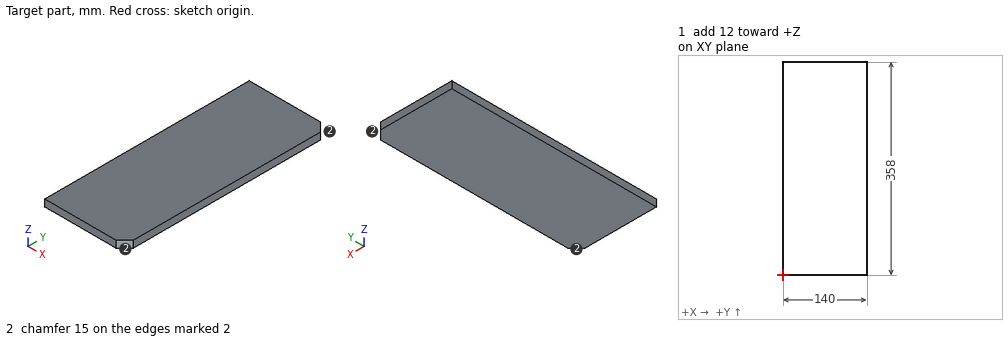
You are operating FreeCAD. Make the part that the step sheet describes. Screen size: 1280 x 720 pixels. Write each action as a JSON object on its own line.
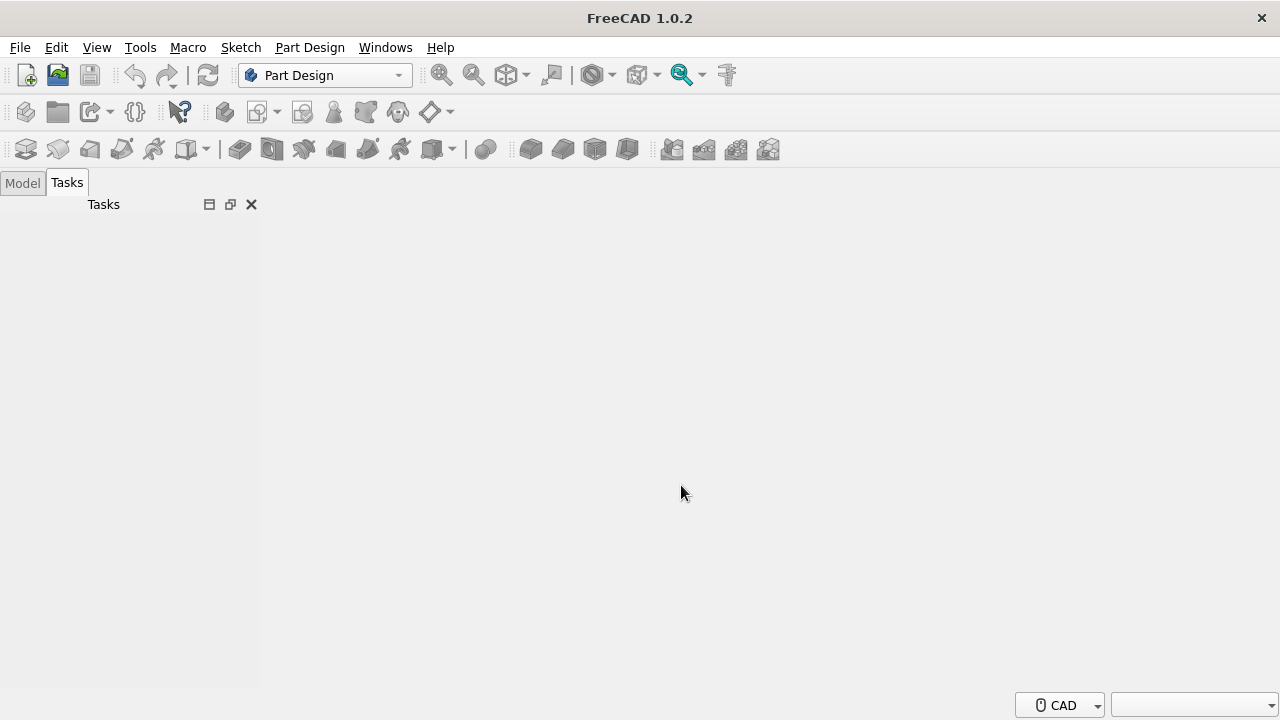
{"action": "left_click", "coordinate": [26, 76]}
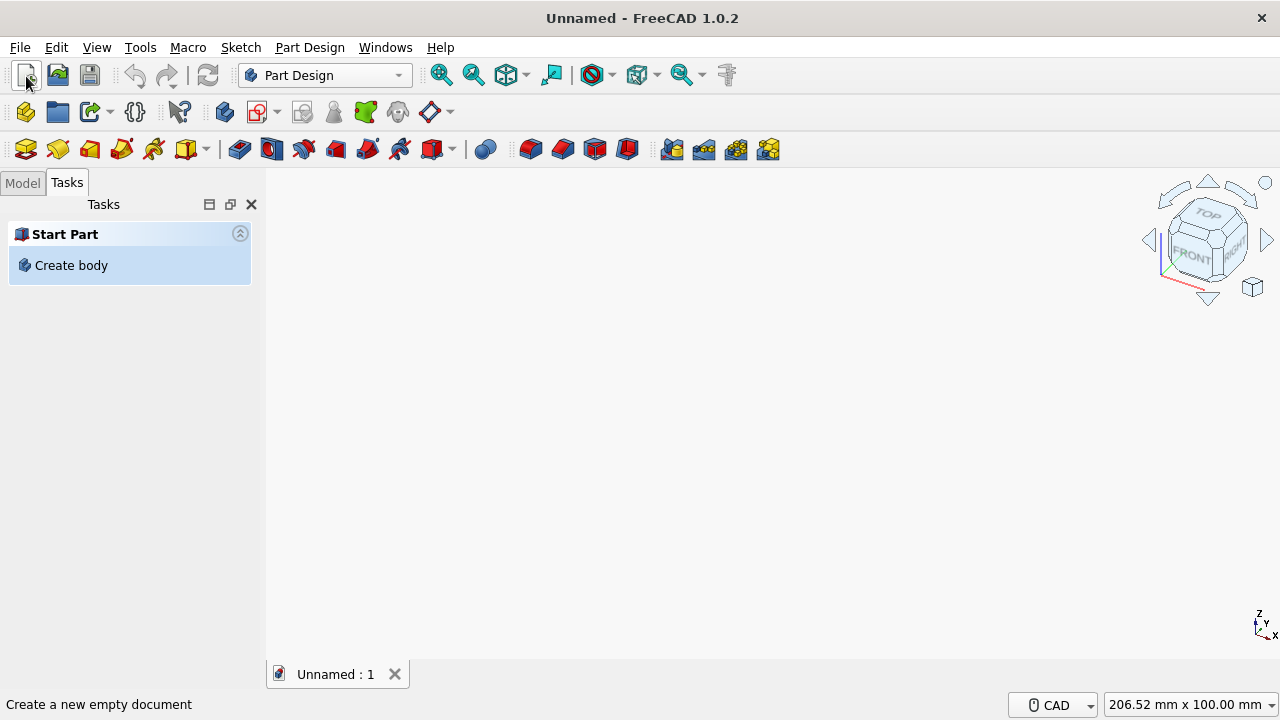
{"action": "left_click", "coordinate": [258, 112]}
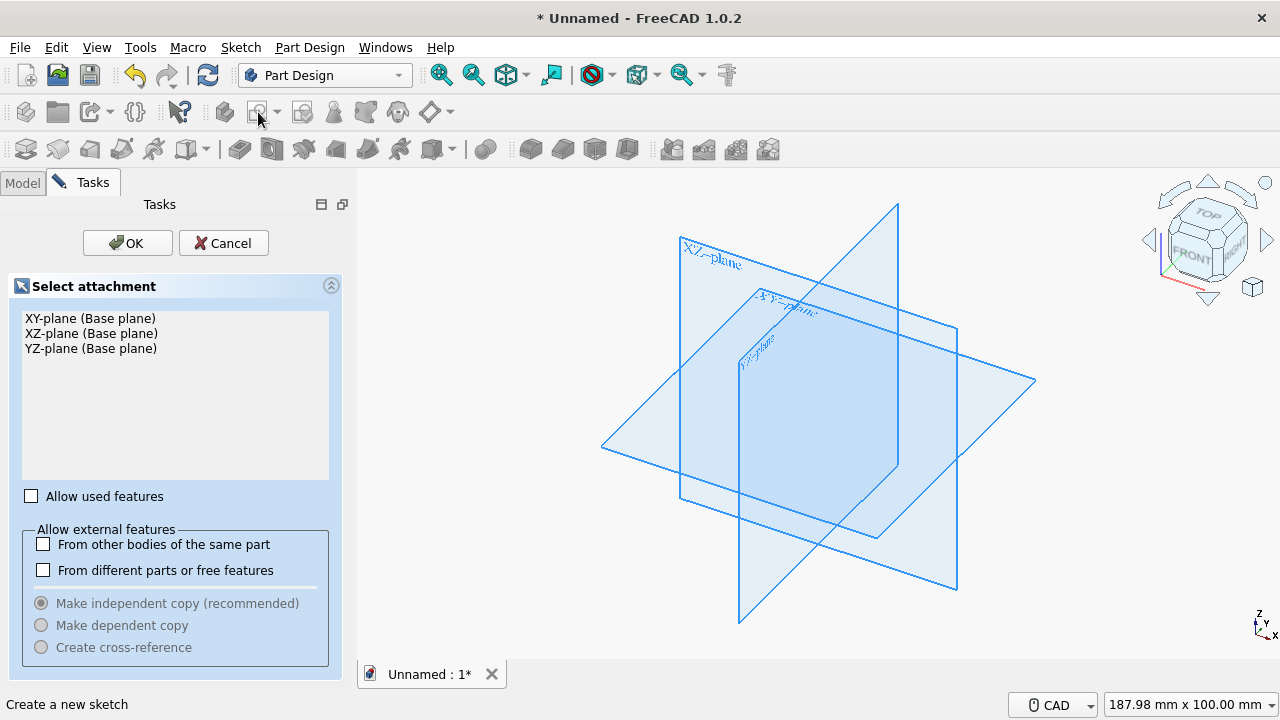
{"action": "left_click", "coordinate": [82, 318]}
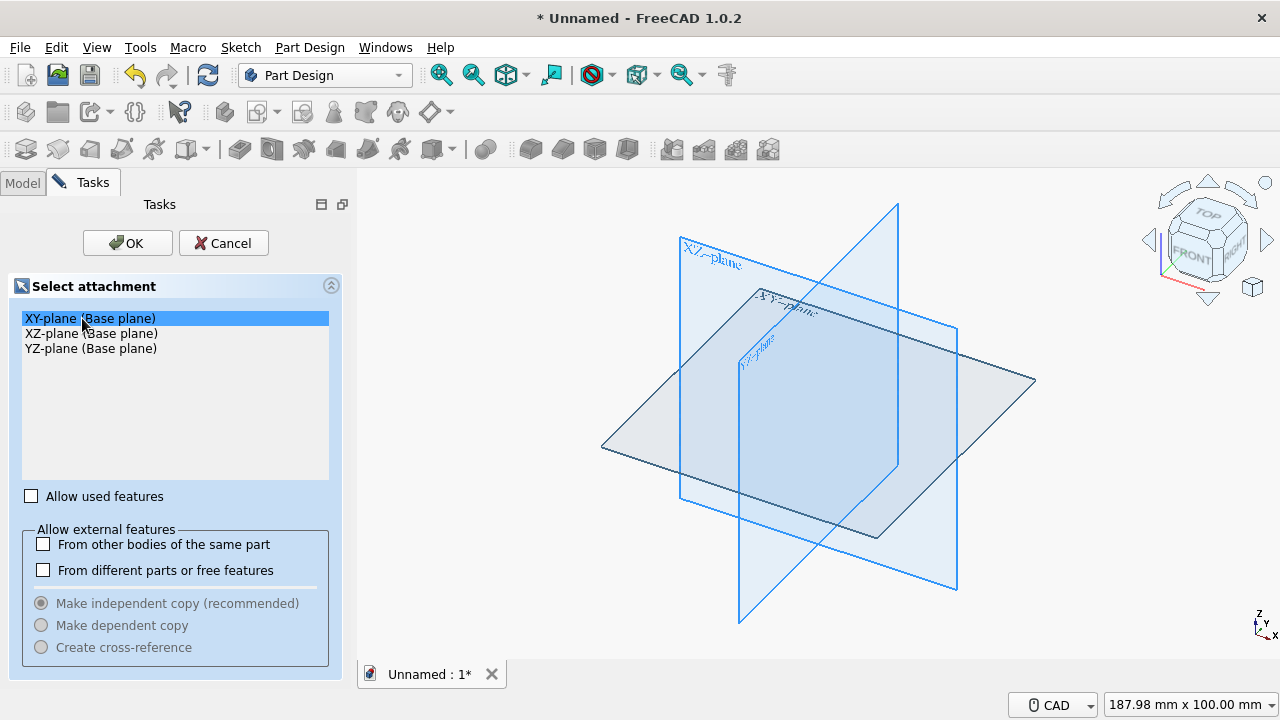
{"action": "left_click", "coordinate": [128, 243]}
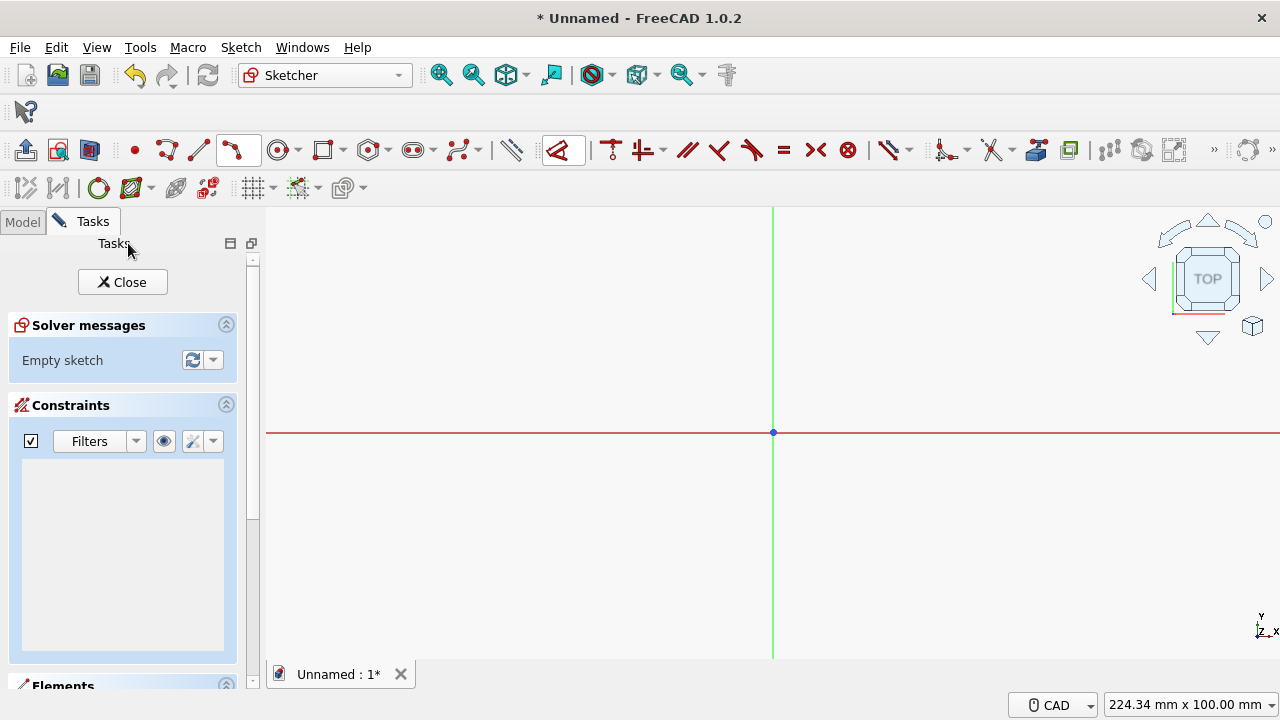
{"action": "scroll", "coordinate": [628, 593], "scroll_direction": "down", "scroll_amount": 9}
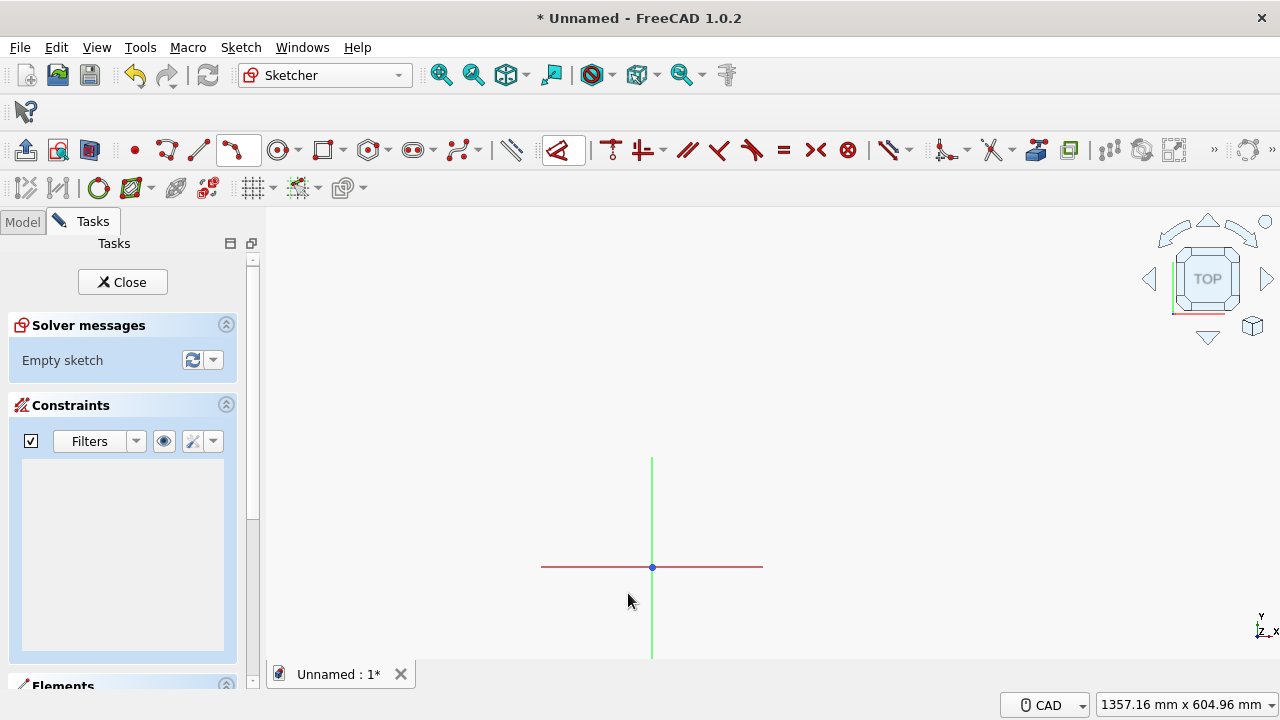
{"action": "left_click", "coordinate": [324, 150]}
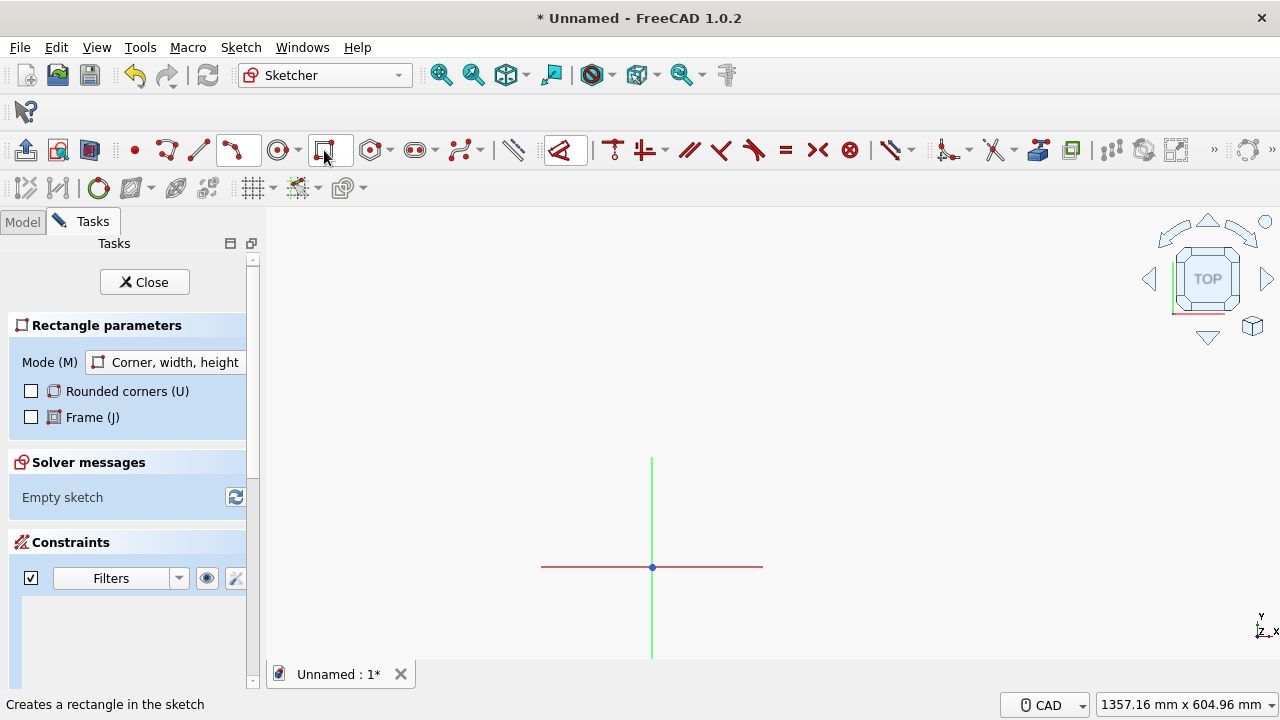
{"action": "left_click", "coordinate": [652, 567]}
{"action": "mouse_move", "coordinate": [757, 300]}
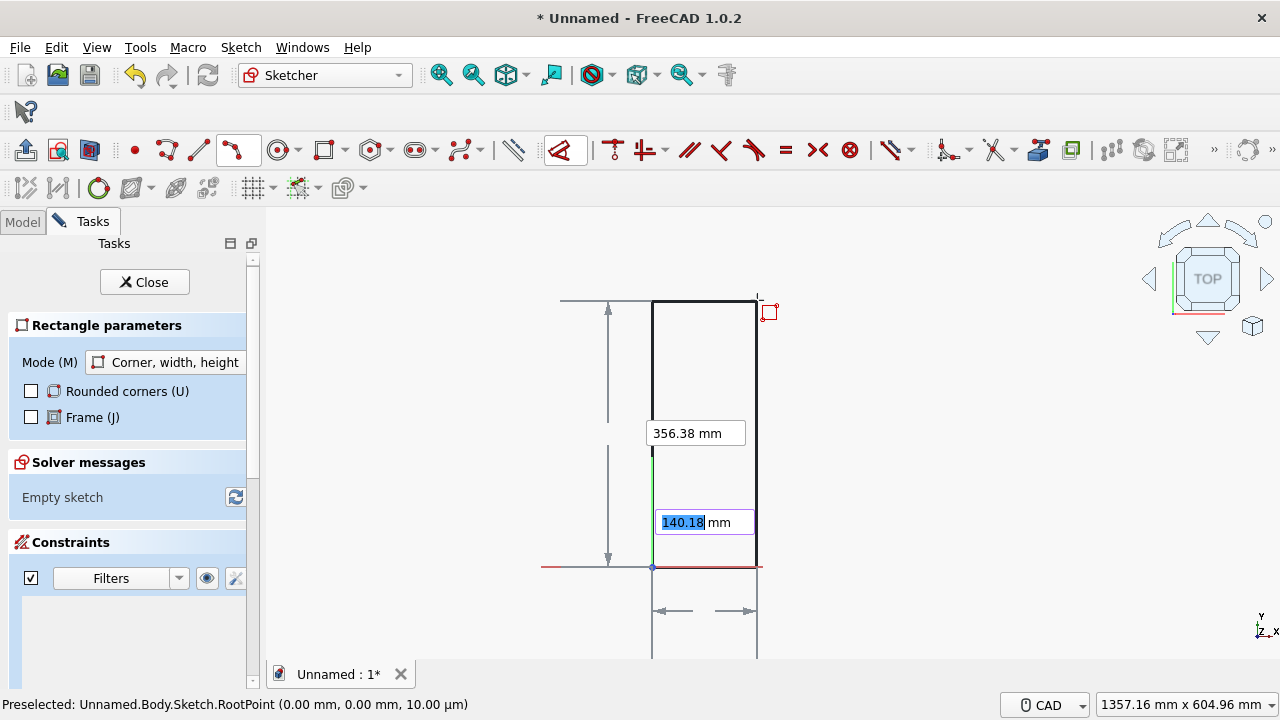
{"action": "type", "text": "140"}
{"action": "key", "text": "Tab"}
{"action": "type", "text": "358"}
{"action": "key", "text": "Return"}
{"action": "key", "text": "Escape"}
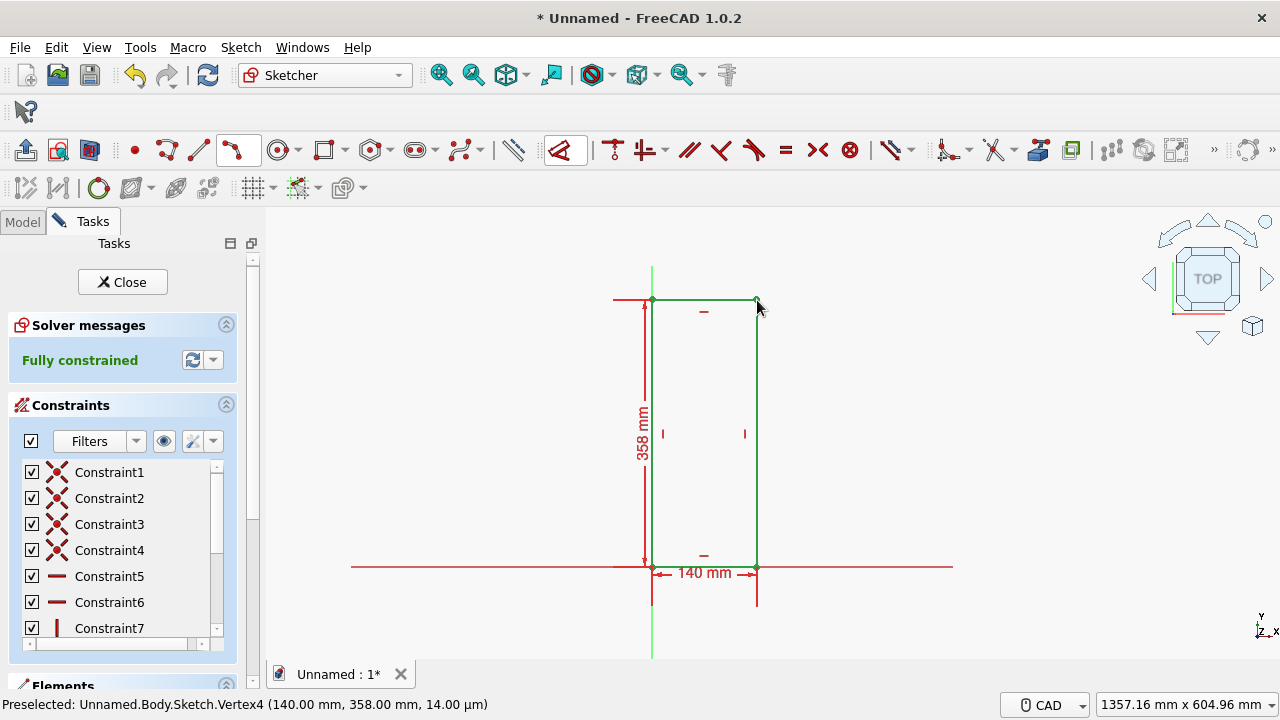
{"action": "left_click", "coordinate": [123, 282]}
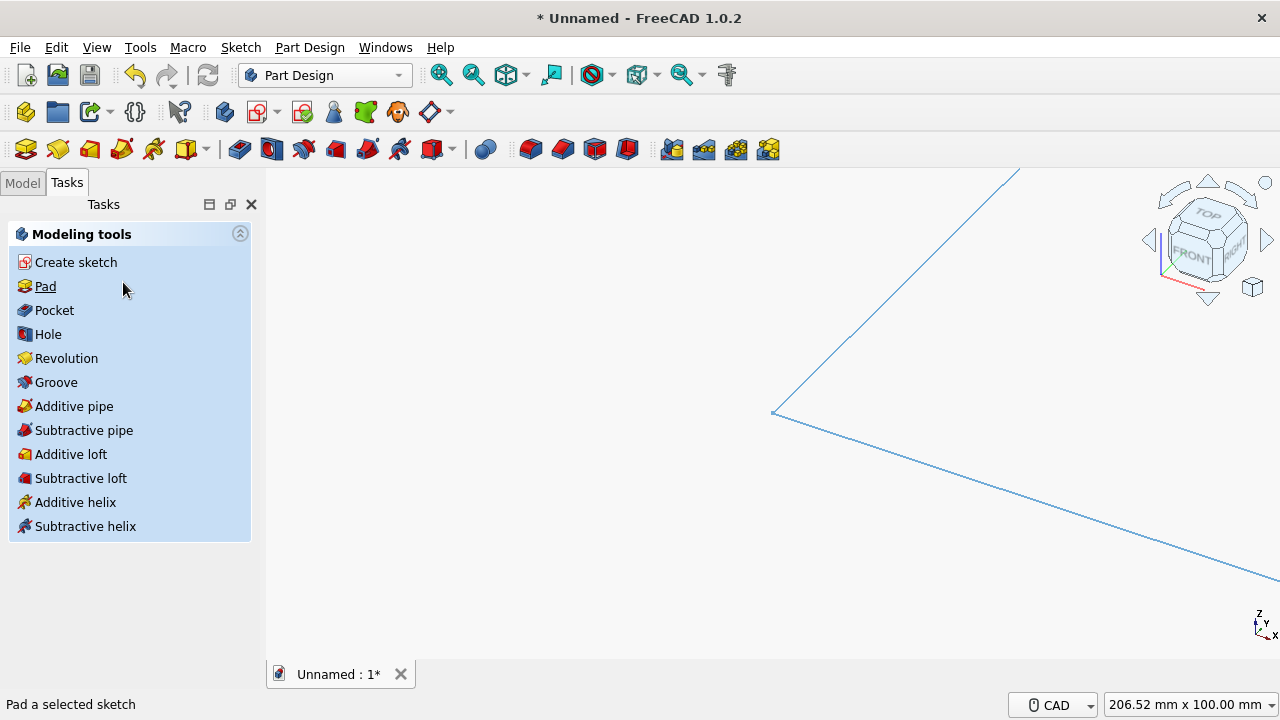
{"action": "left_click", "coordinate": [26, 150]}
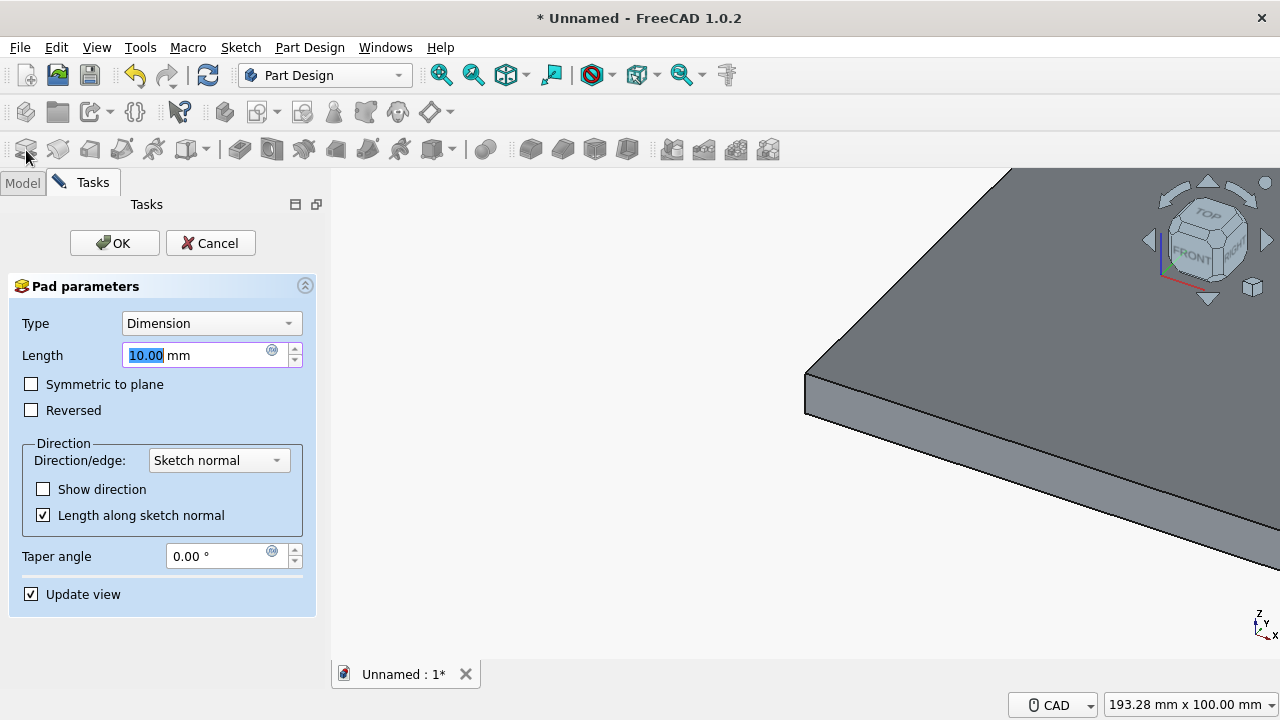
{"action": "type", "text": "12"}
{"action": "key", "text": "Tab"}